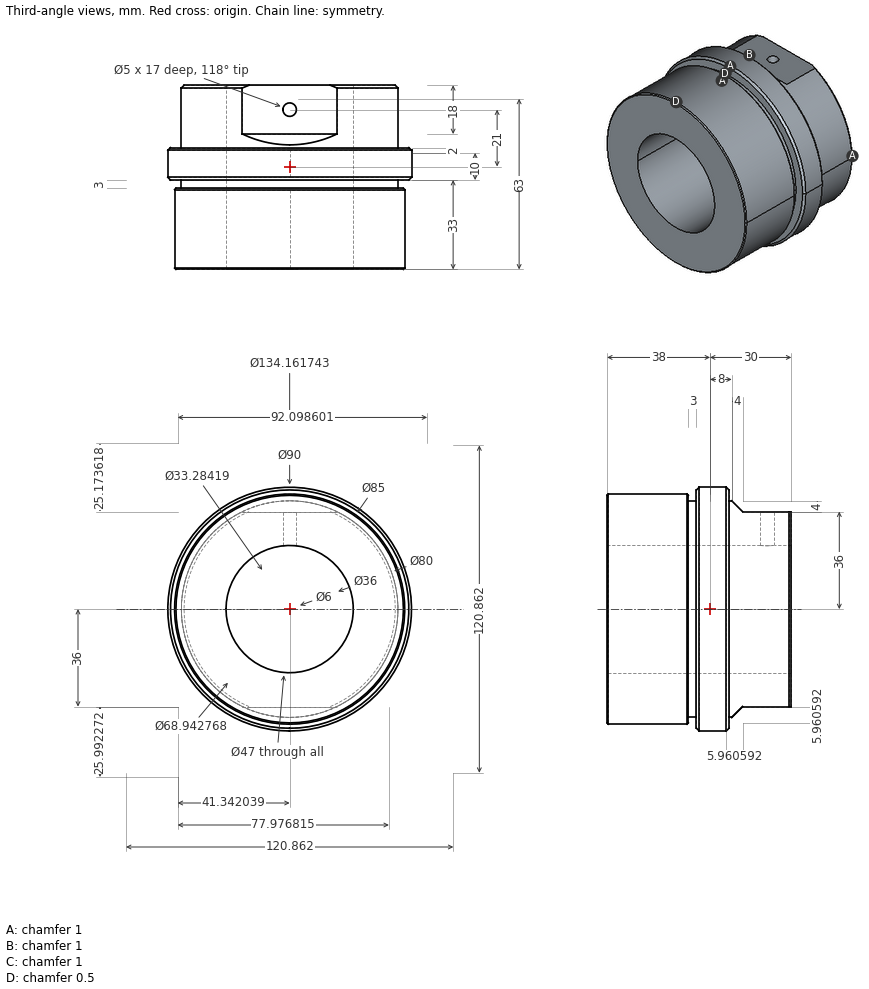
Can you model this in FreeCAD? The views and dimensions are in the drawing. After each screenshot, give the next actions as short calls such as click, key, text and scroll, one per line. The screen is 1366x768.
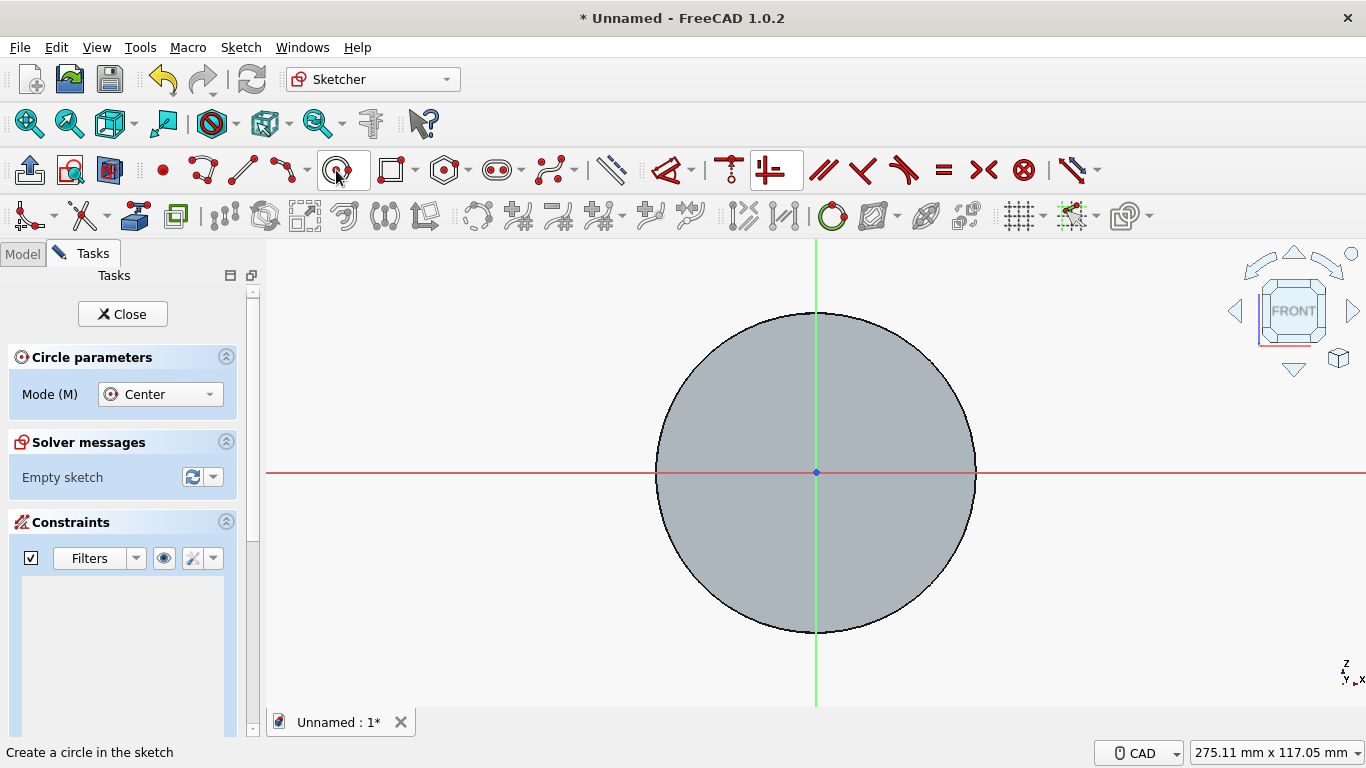
click(816, 473)
click(936, 353)
key(Escape)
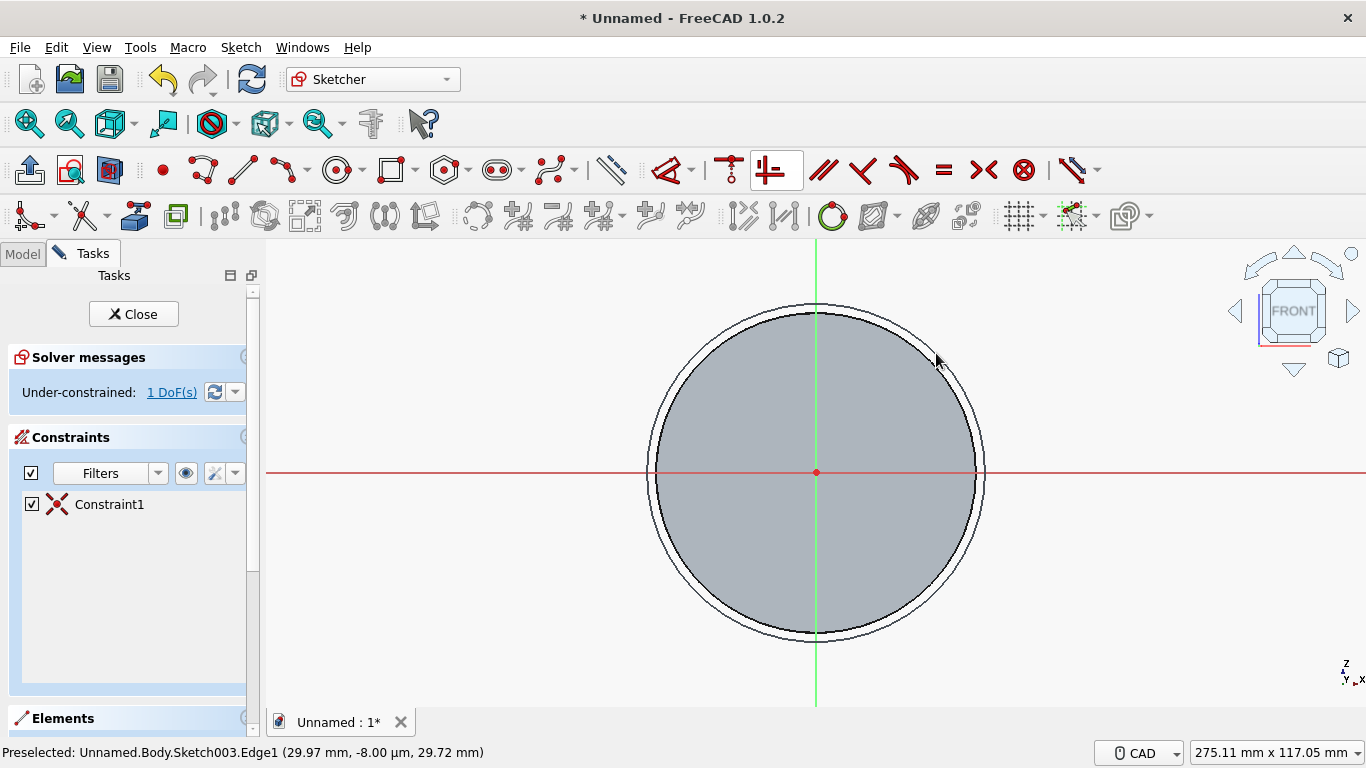
click(666, 170)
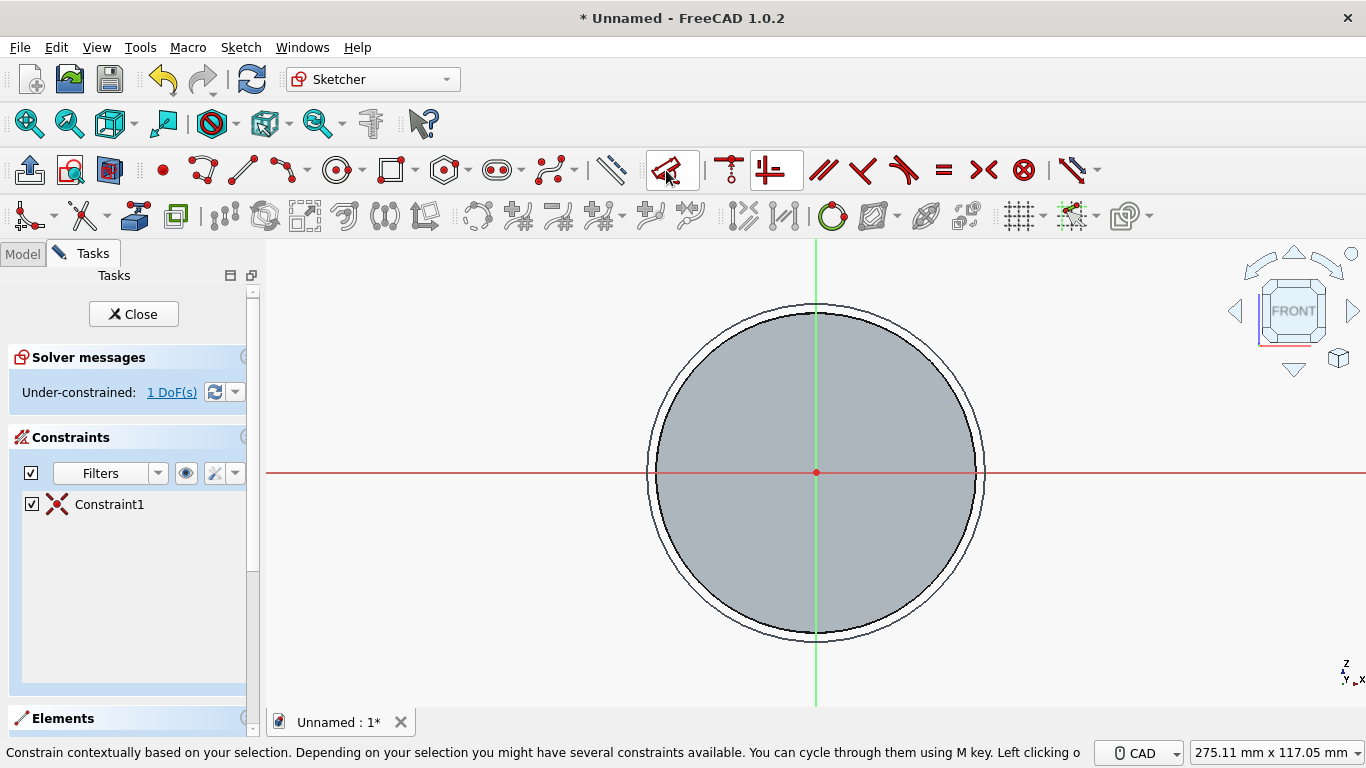
click(935, 353)
click(958, 330)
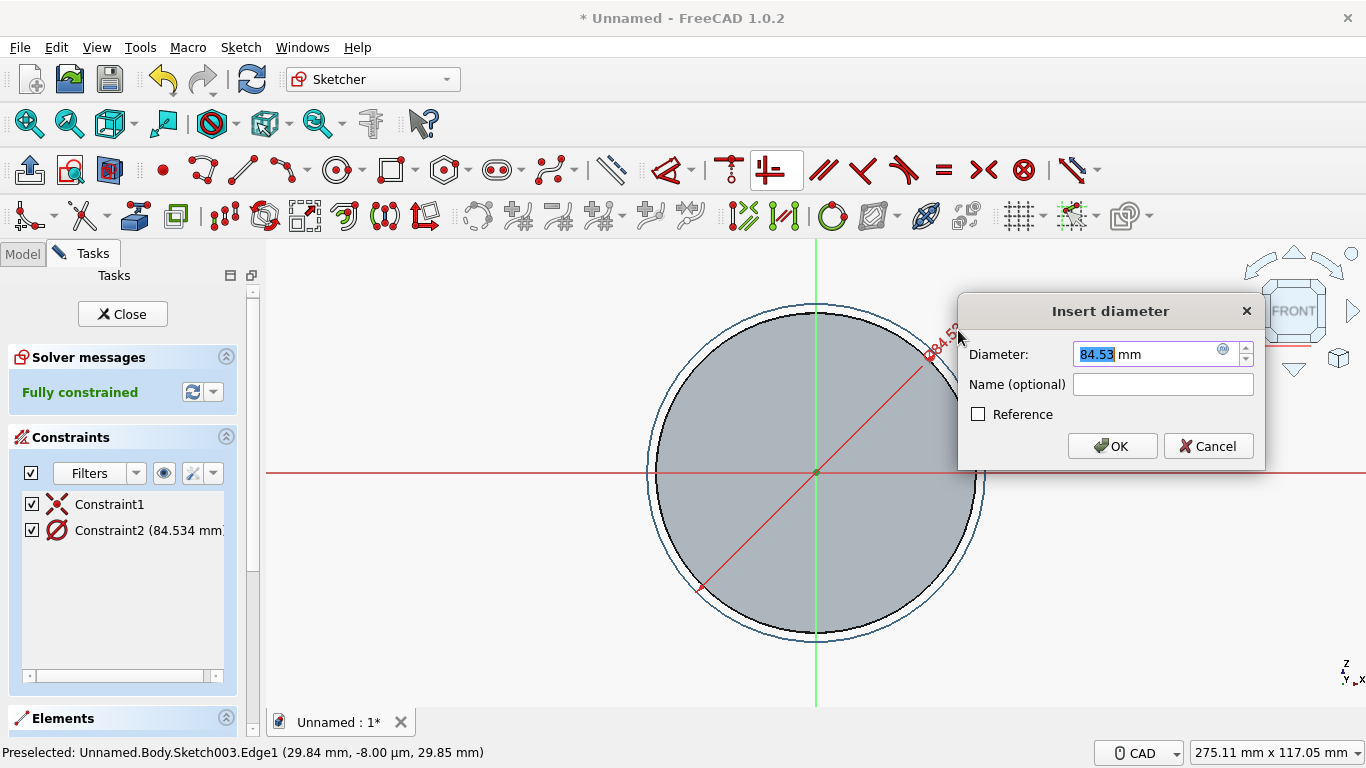
text(85)
key(Return)
key(Escape)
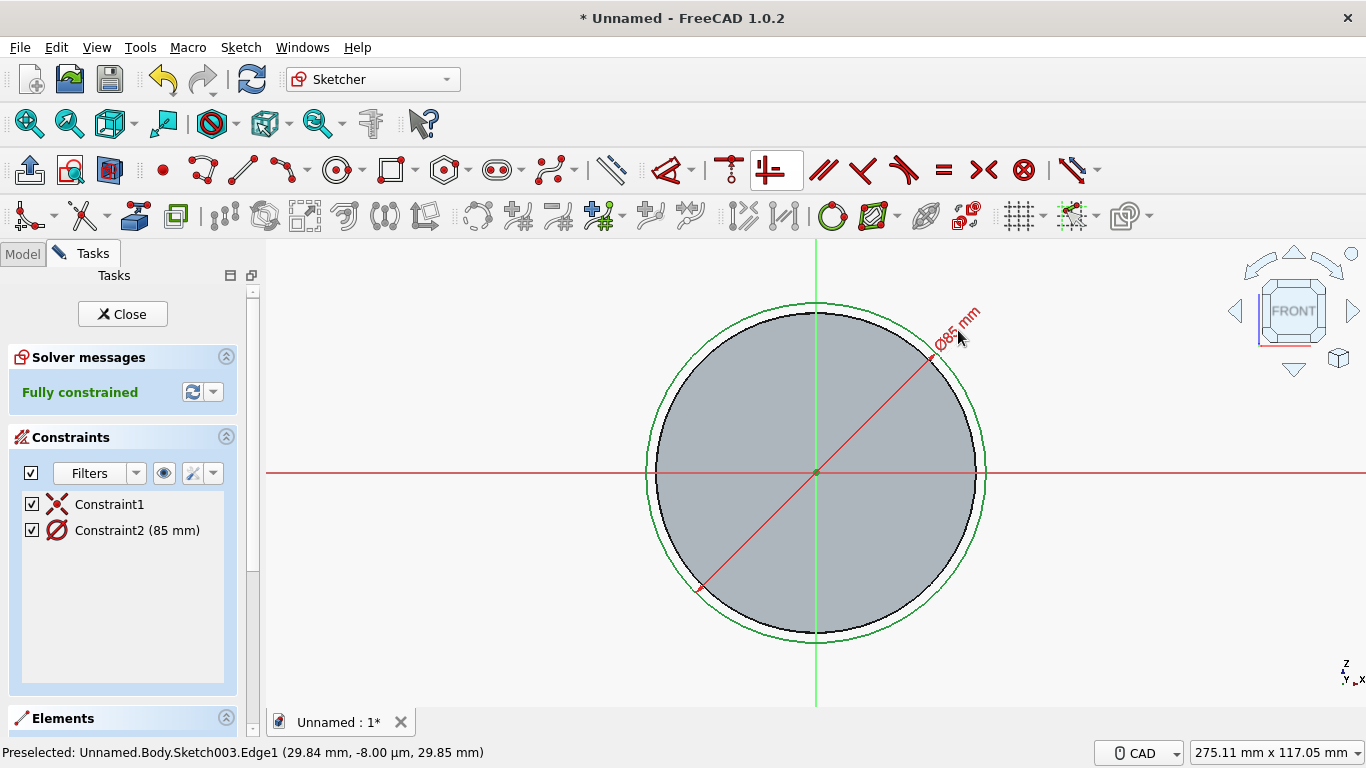
click(123, 314)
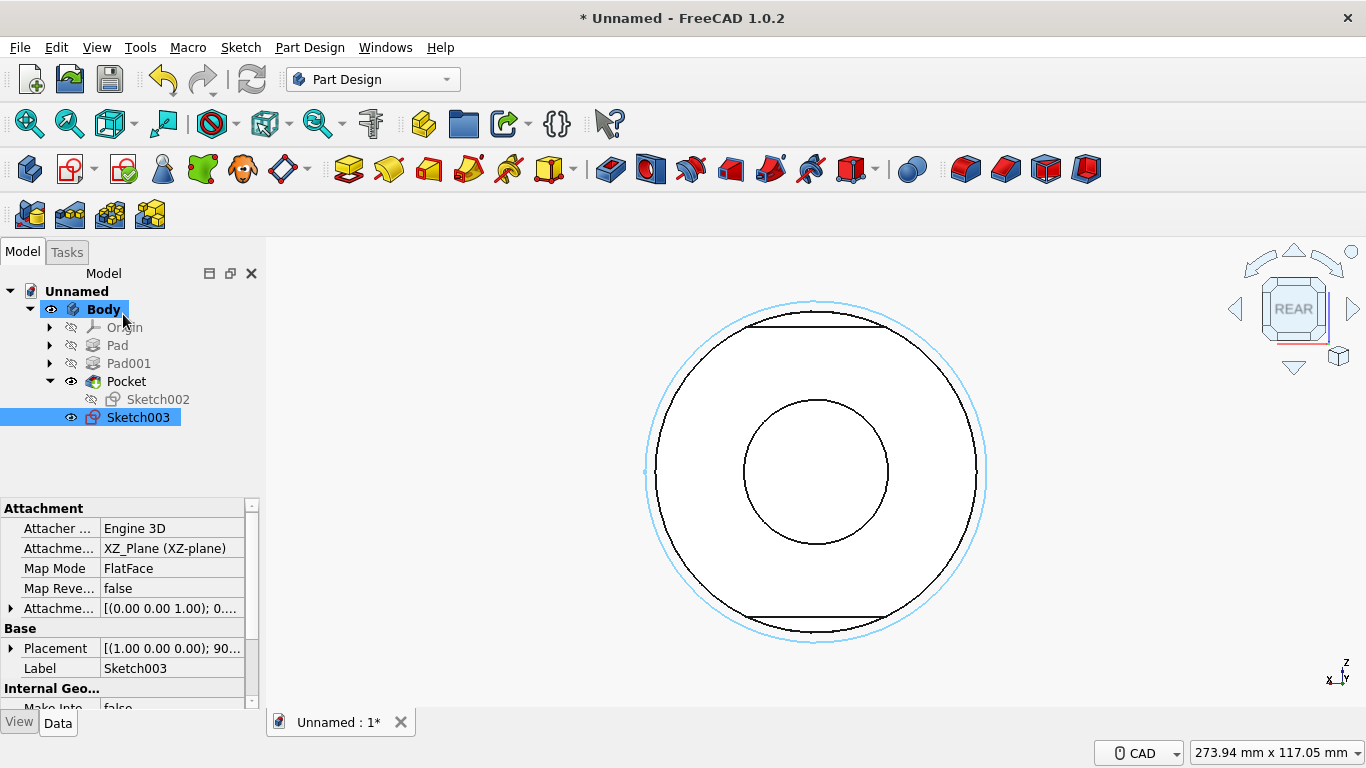
click(350, 170)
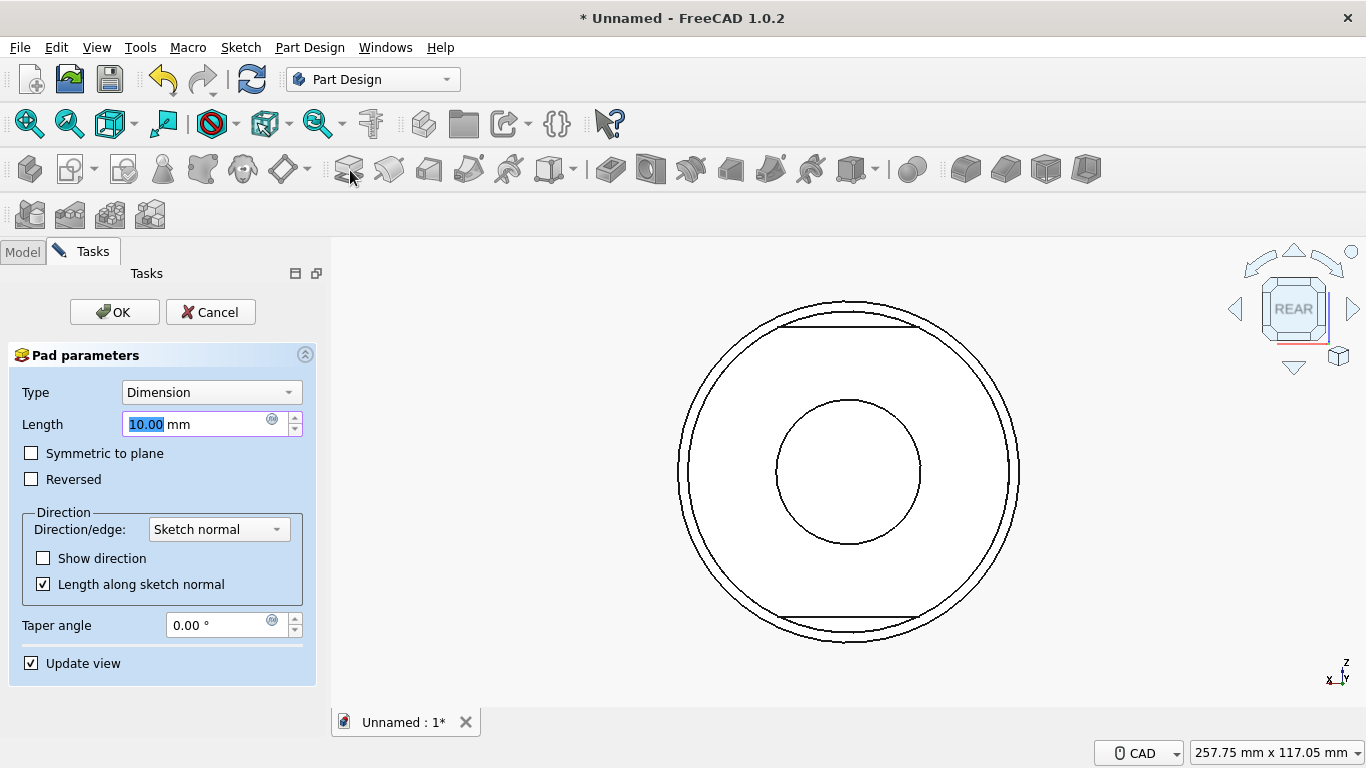
text(38)
key(Tab)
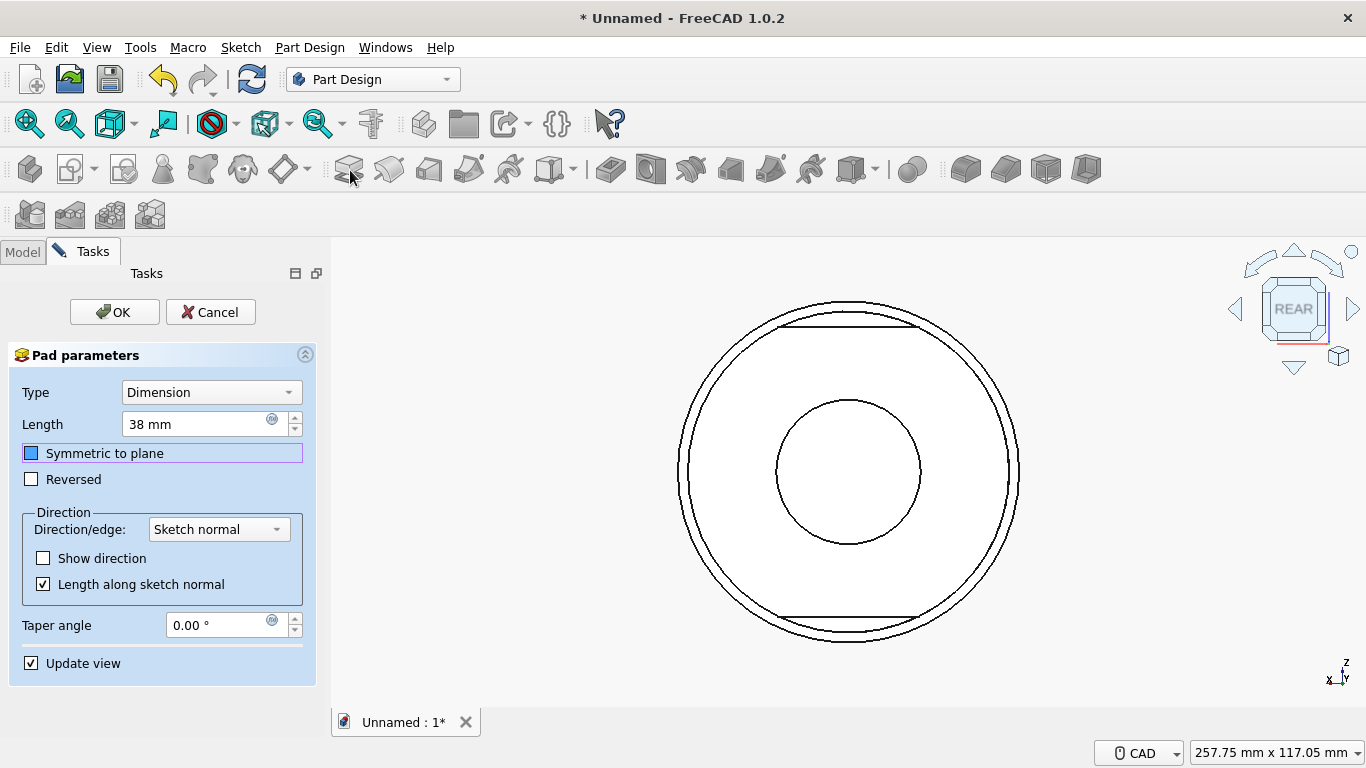
click(115, 312)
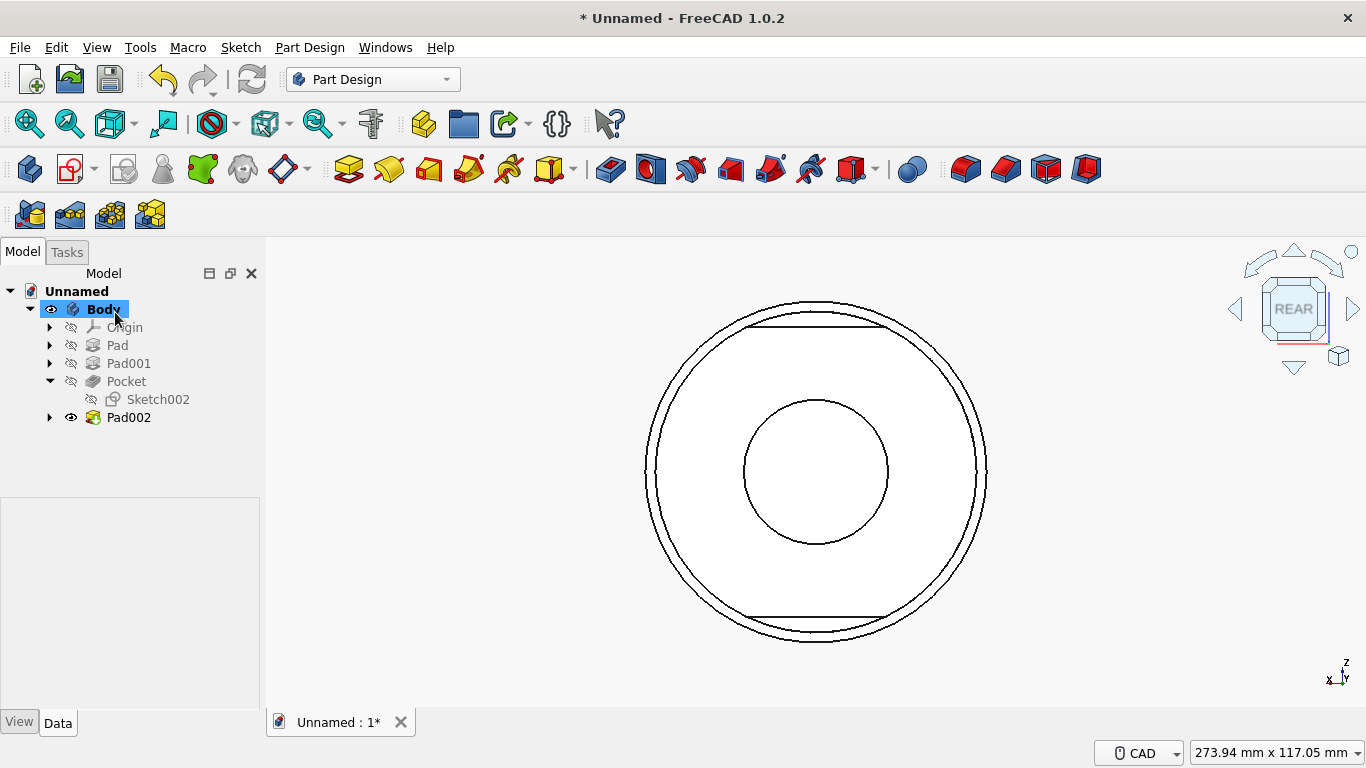
key(0)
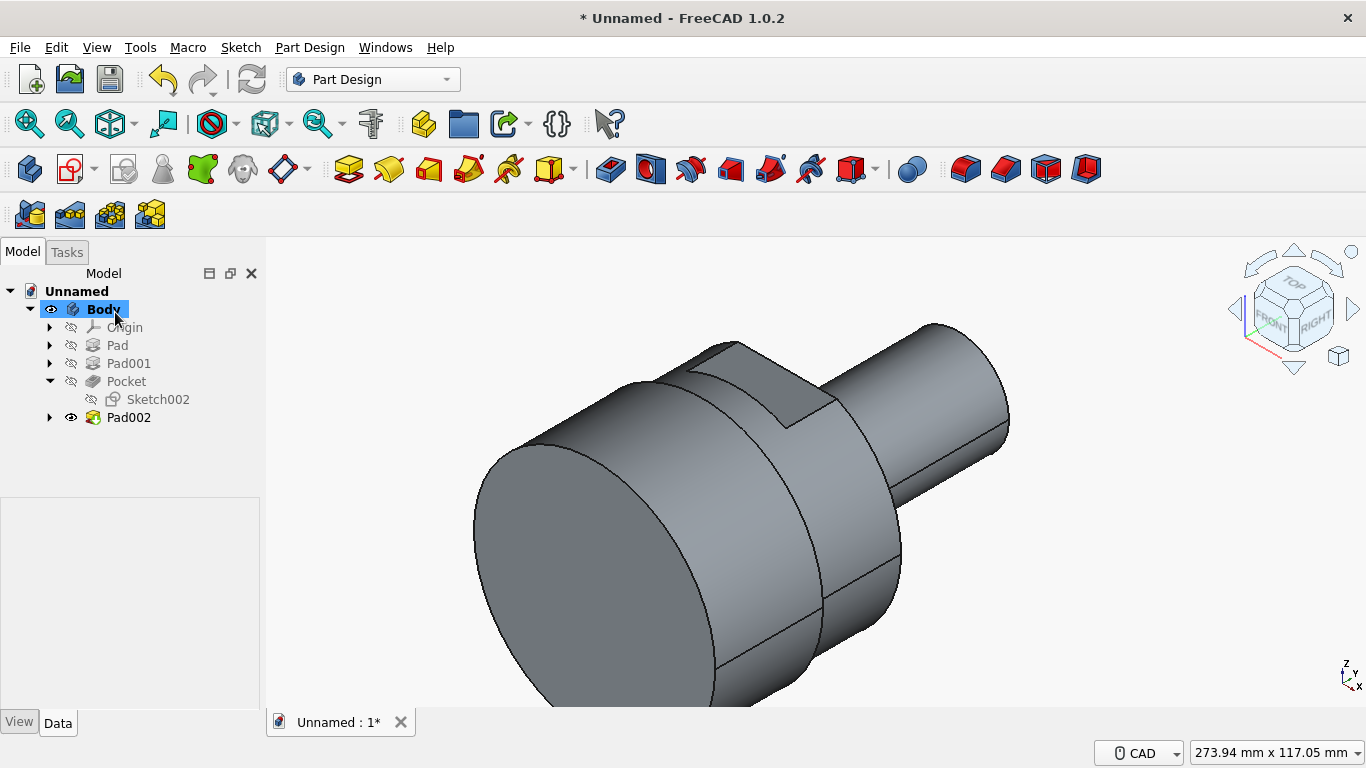
click(30, 124)